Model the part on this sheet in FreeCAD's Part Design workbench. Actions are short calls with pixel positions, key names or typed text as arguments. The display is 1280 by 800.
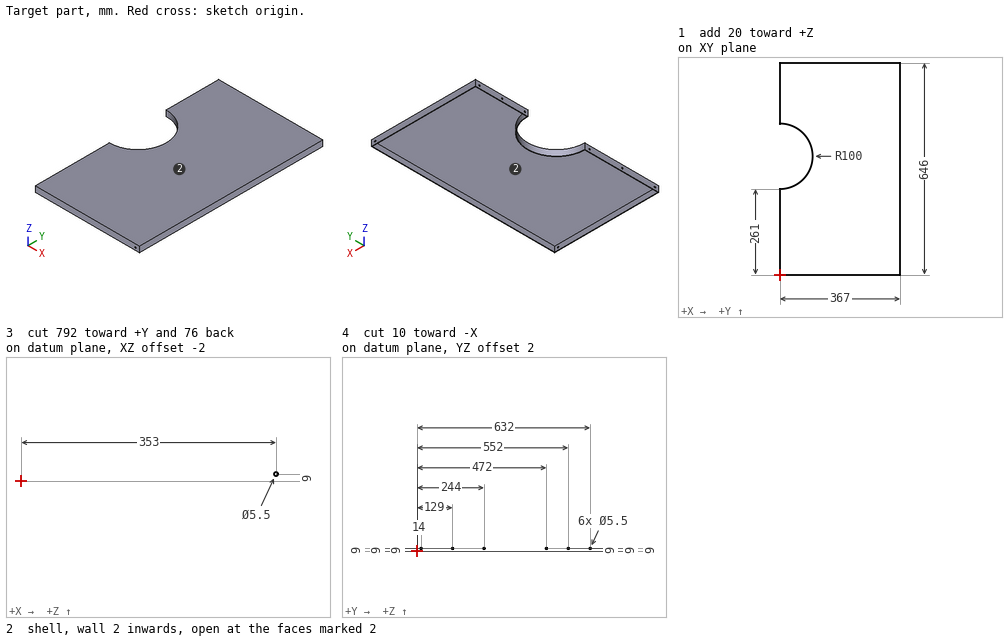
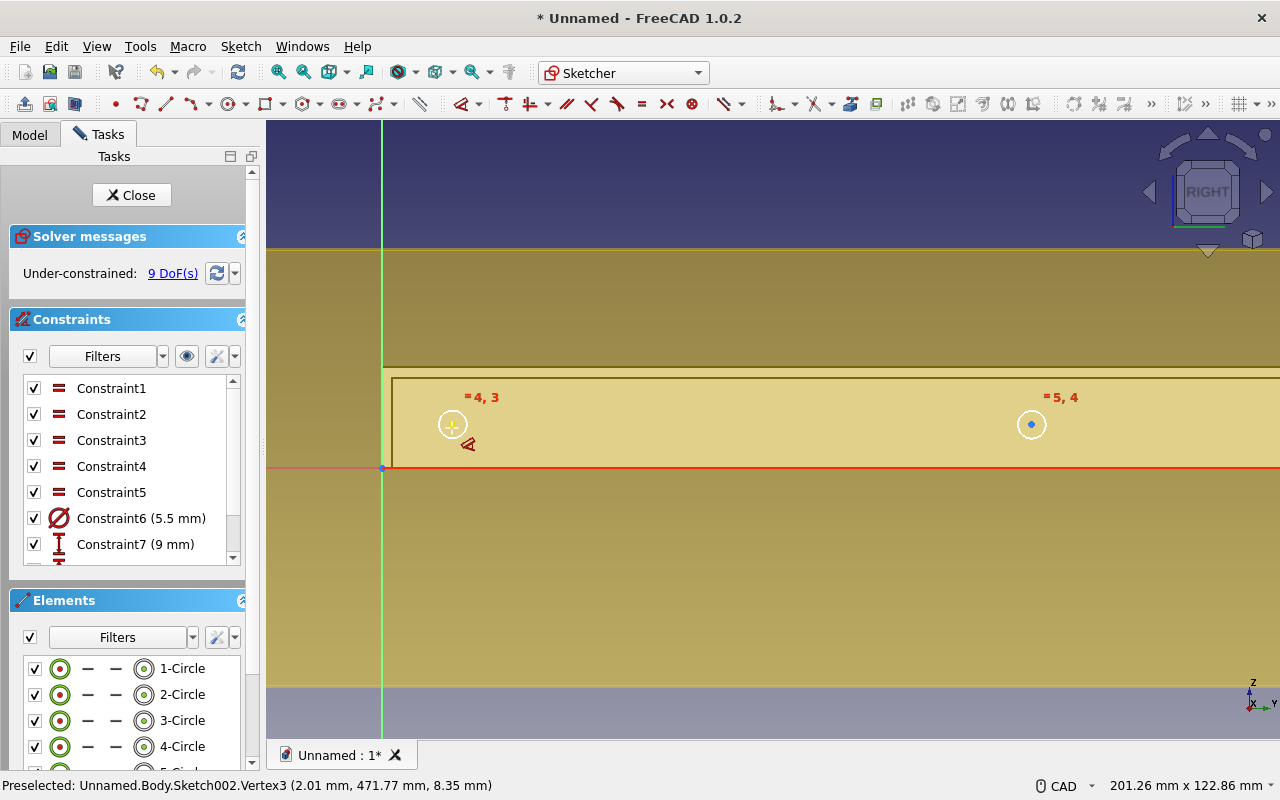
click(453, 424)
click(348, 446)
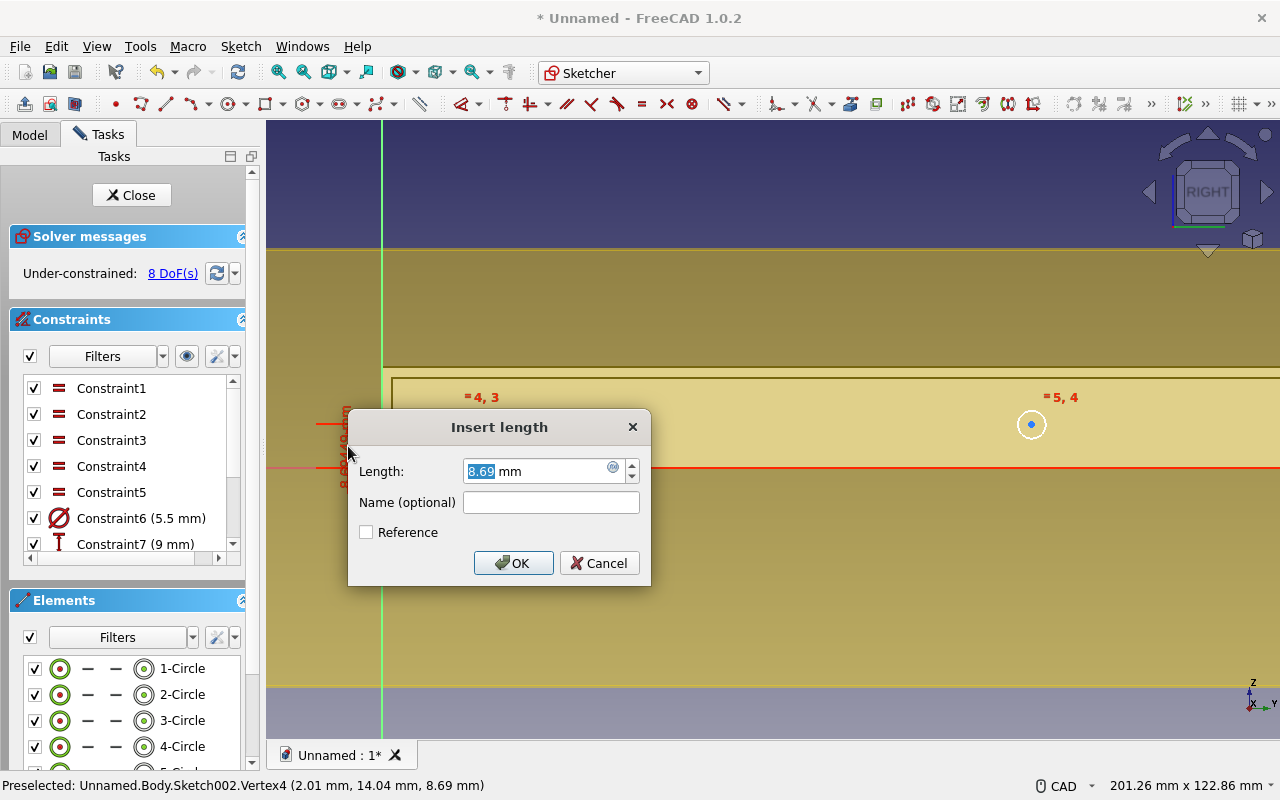
text(9)
key(Return)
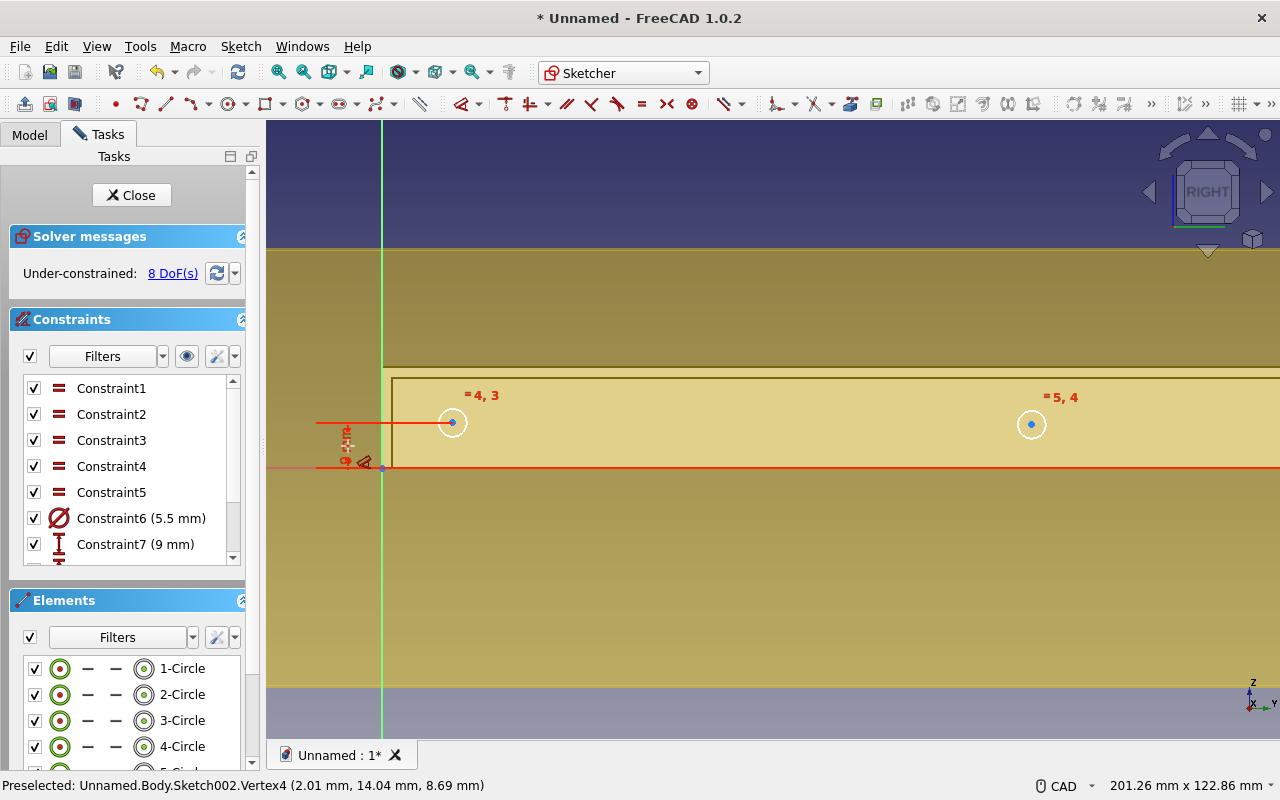
click(1032, 425)
click(1066, 446)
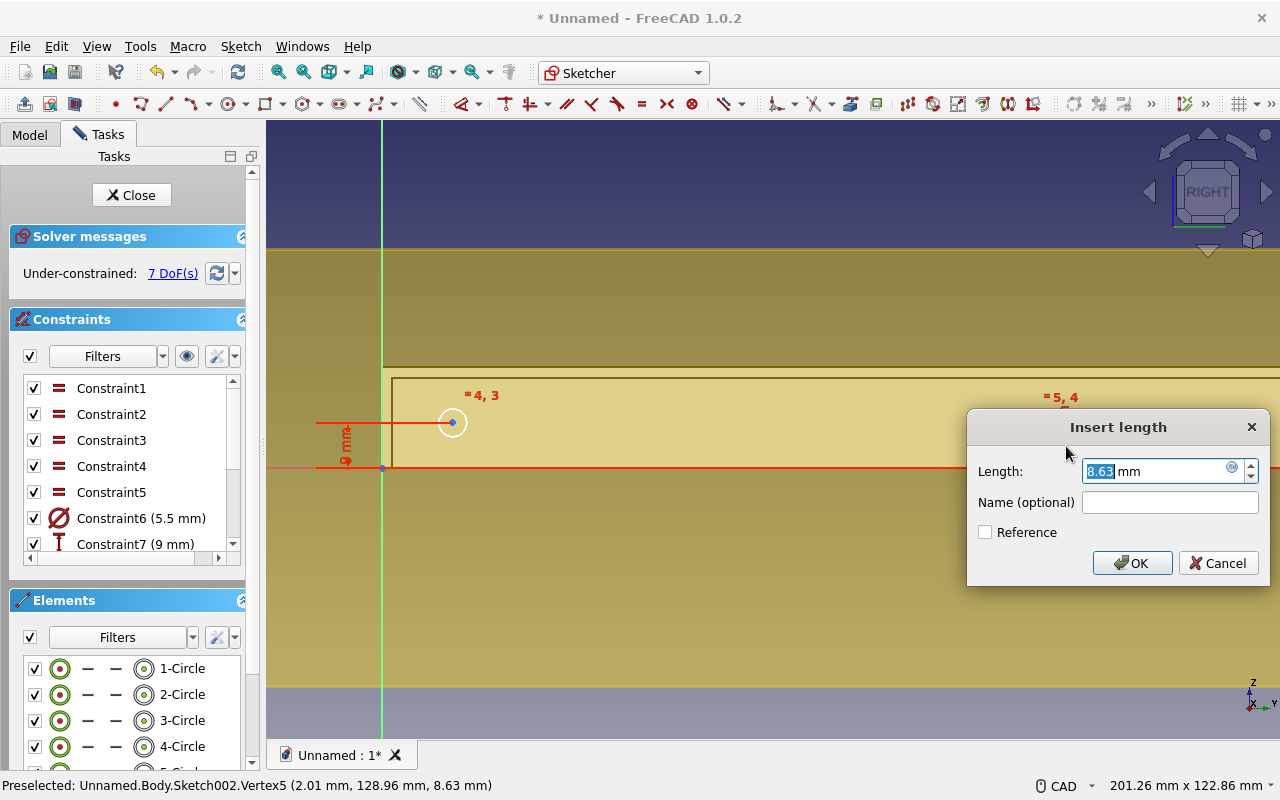
text(9)
key(Return)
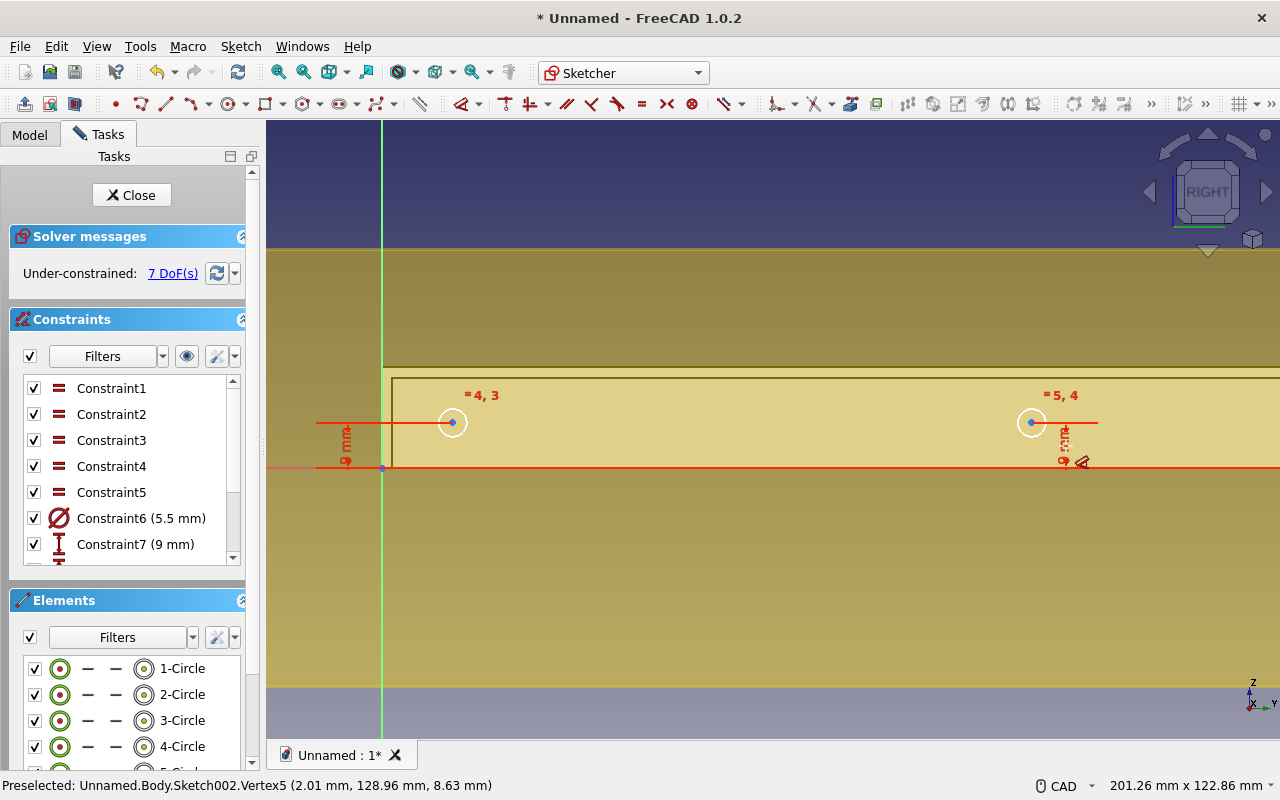
scroll(452, 428, down, 9)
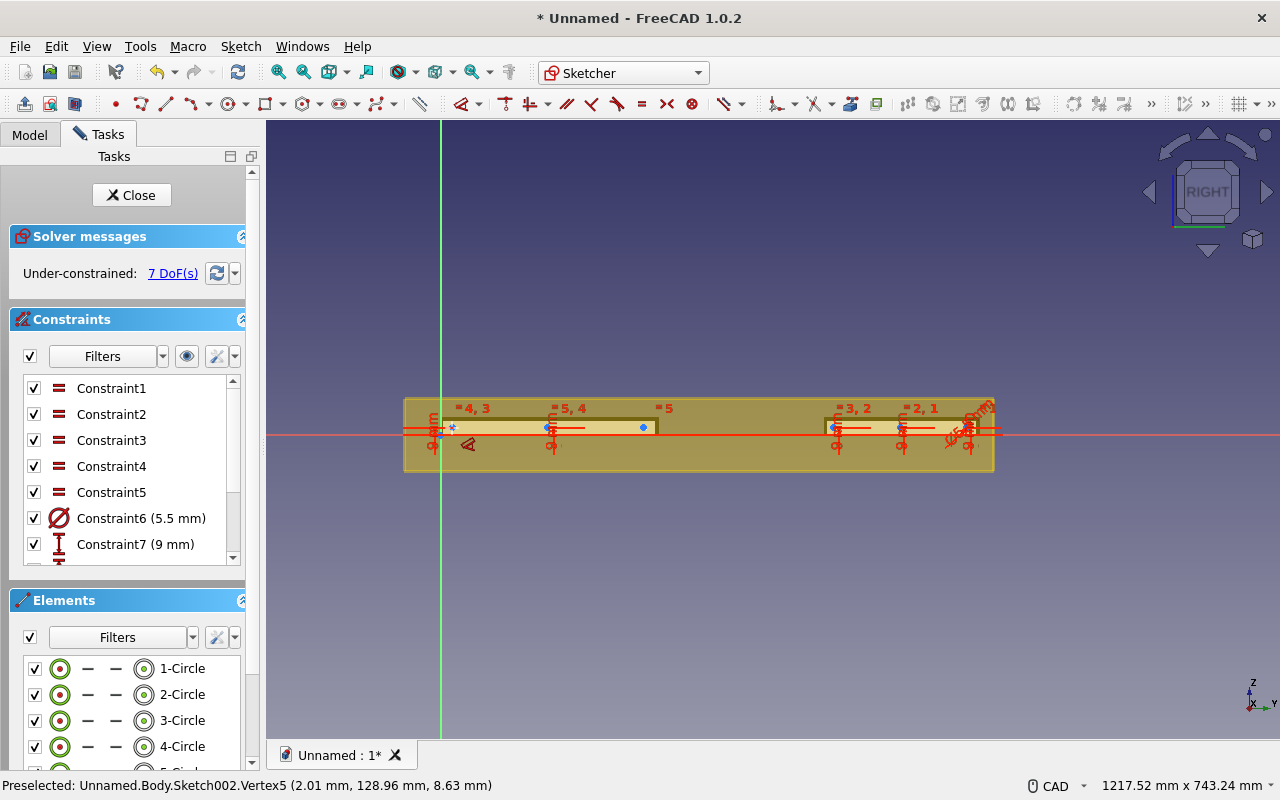
scroll(644, 428, up, 9)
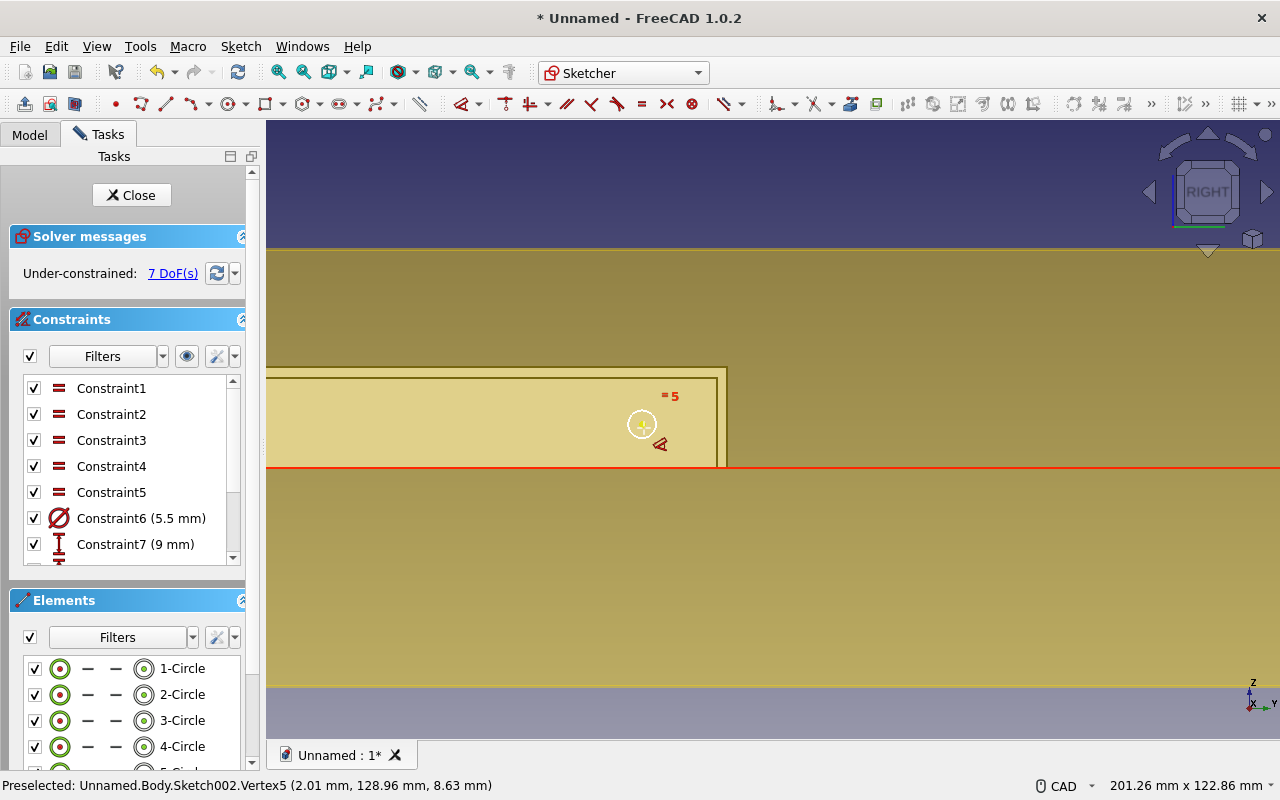
click(642, 424)
click(676, 446)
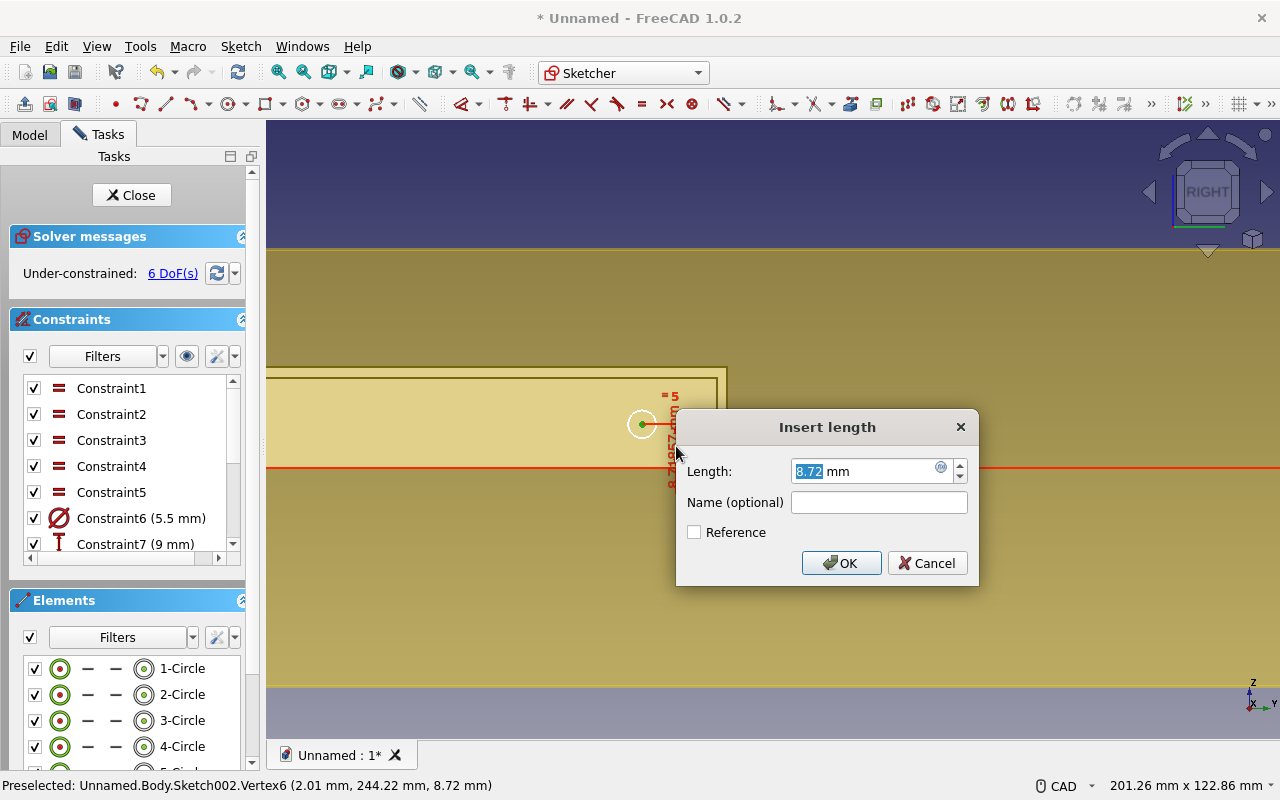
text(9)
key(Return)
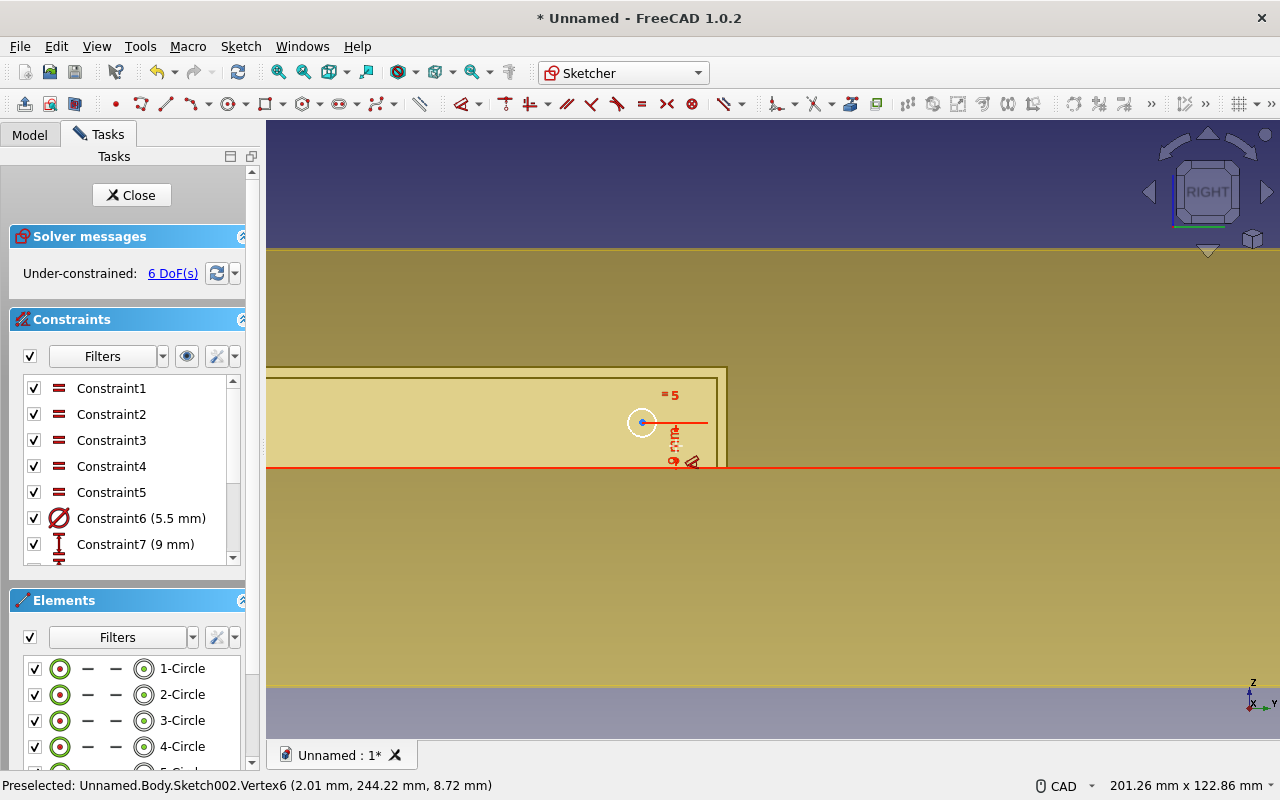
scroll(644, 428, down, 9)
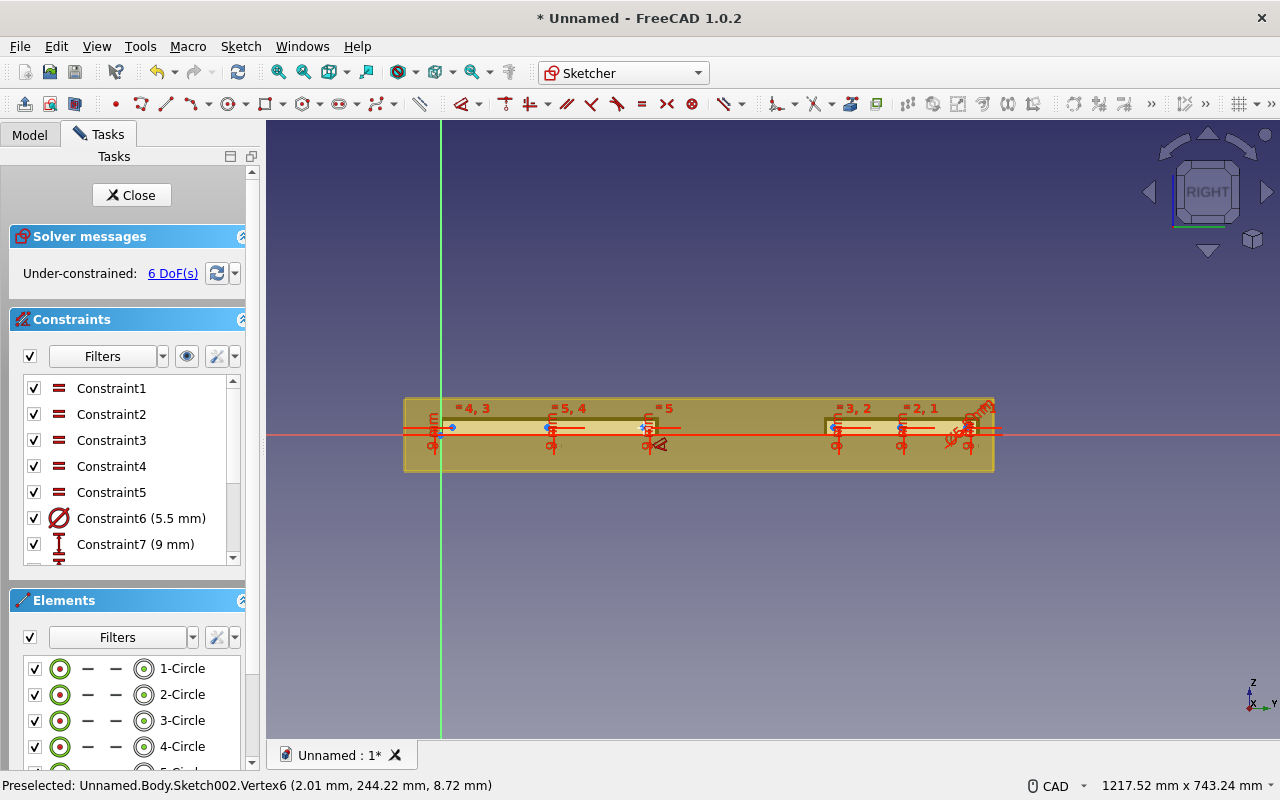
scroll(452, 428, up, 7)